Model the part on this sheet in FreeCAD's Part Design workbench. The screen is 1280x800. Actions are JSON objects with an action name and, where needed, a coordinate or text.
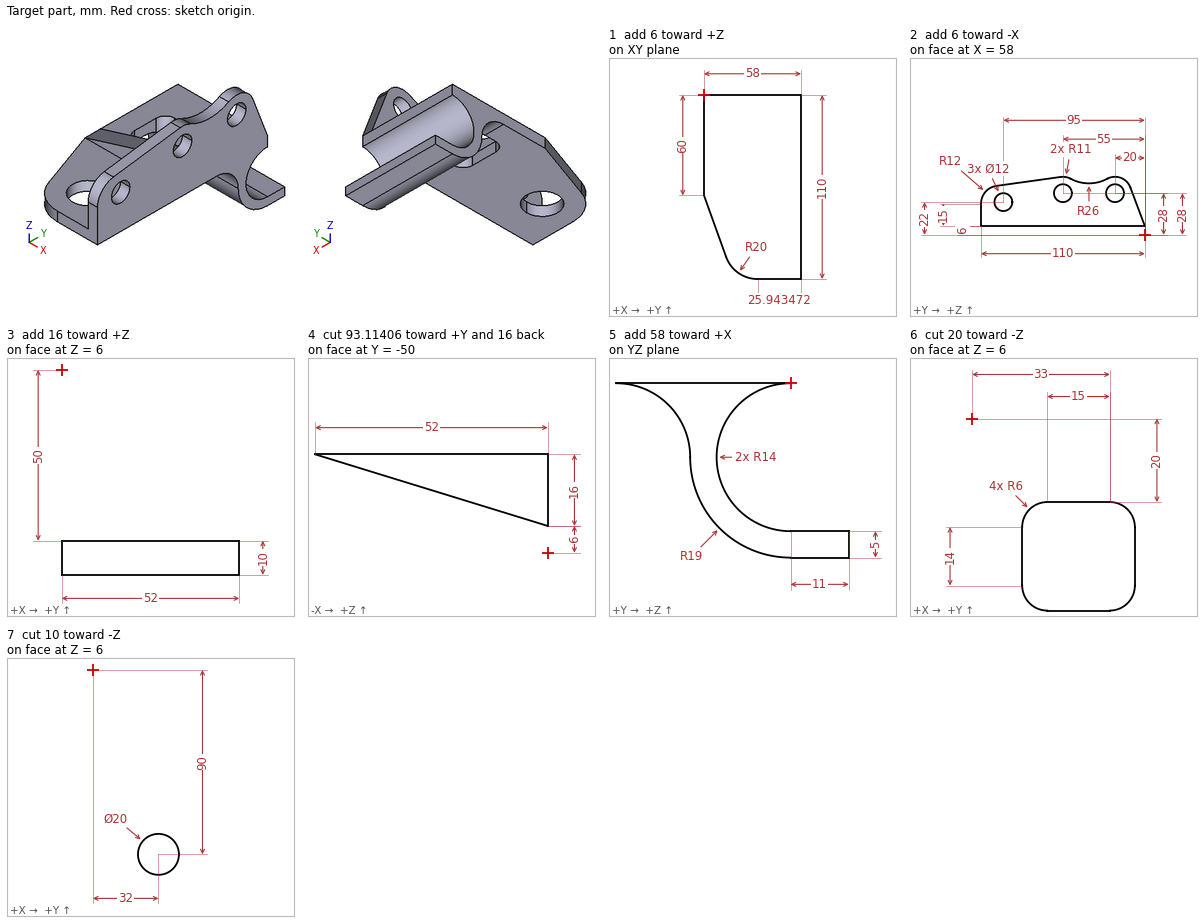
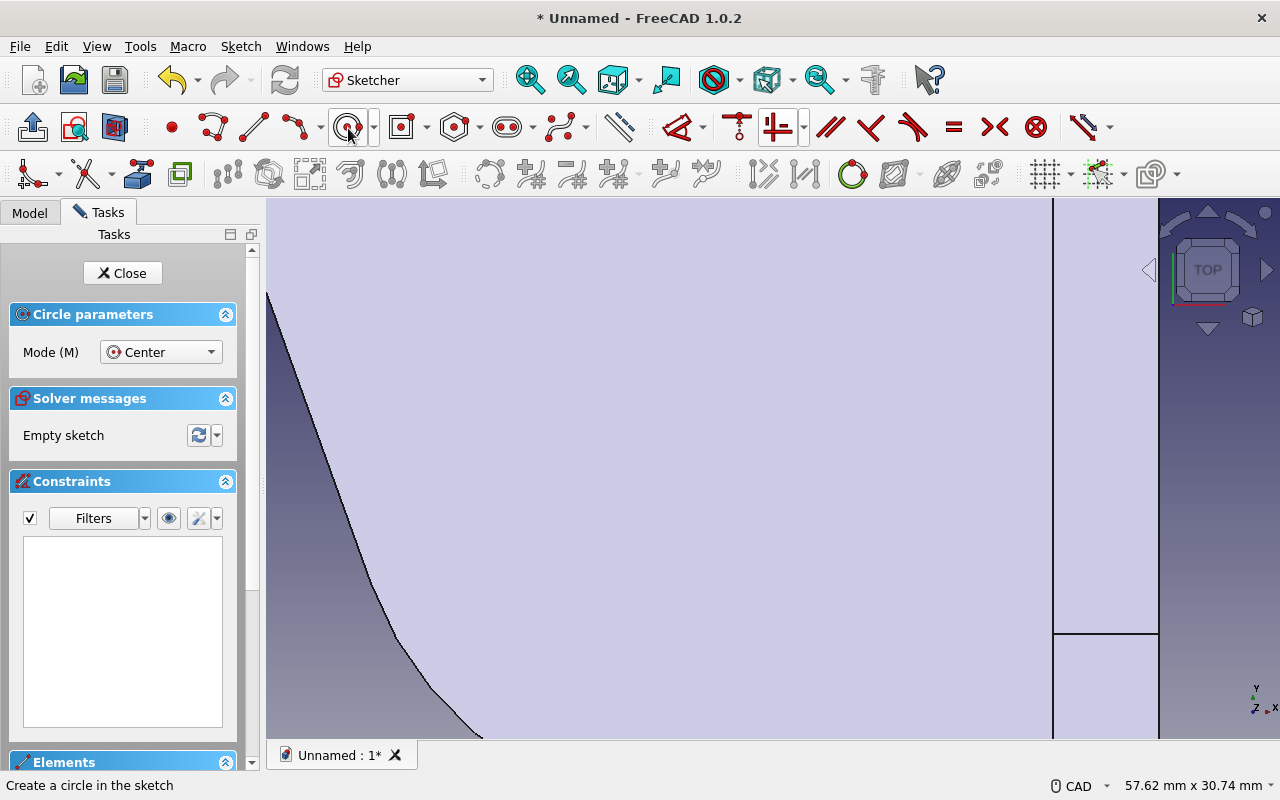
{"action": "left_click", "coordinate": [701, 464]}
{"action": "mouse_move", "coordinate": [826, 340]}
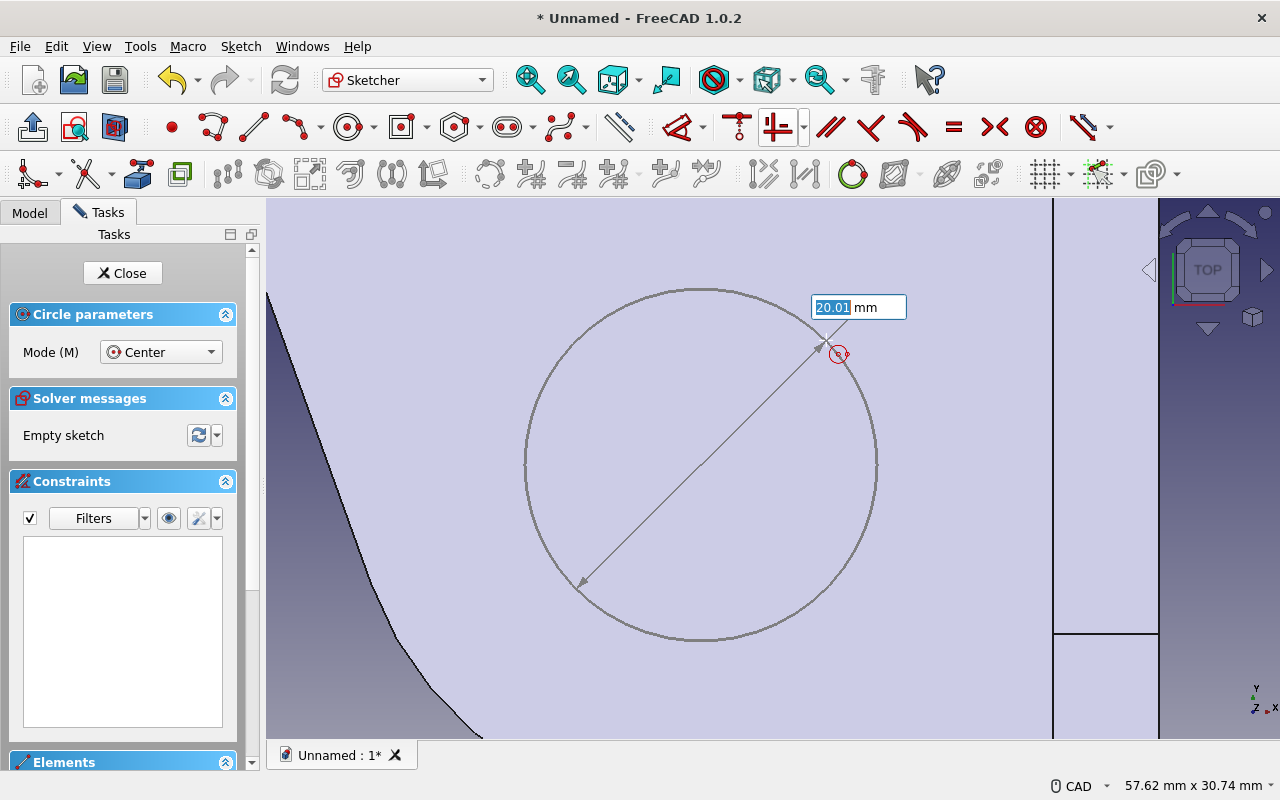
{"action": "type", "text": "20"}
{"action": "key", "text": "Return"}
{"action": "key", "text": "Escape"}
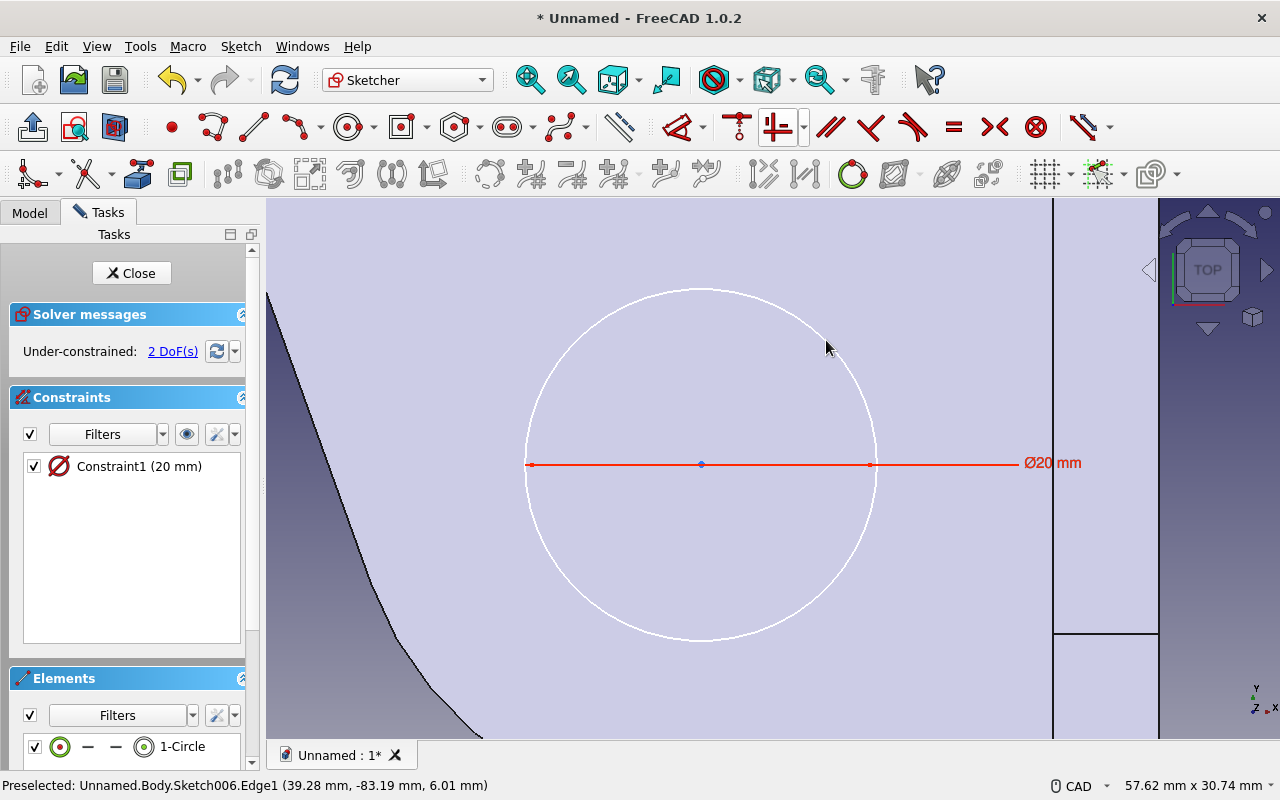
{"action": "key", "text": "d"}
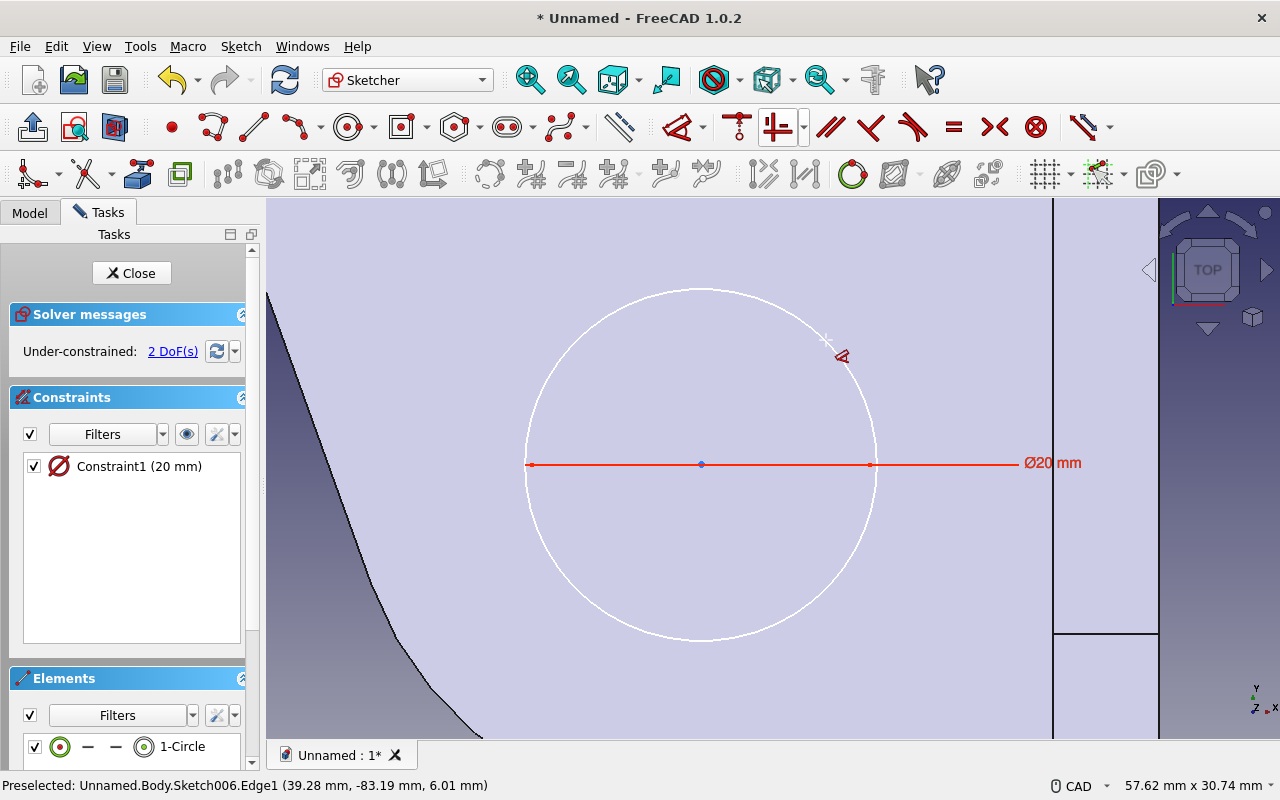
{"action": "left_click", "coordinate": [701, 465]}
{"action": "left_click", "coordinate": [498, 499]}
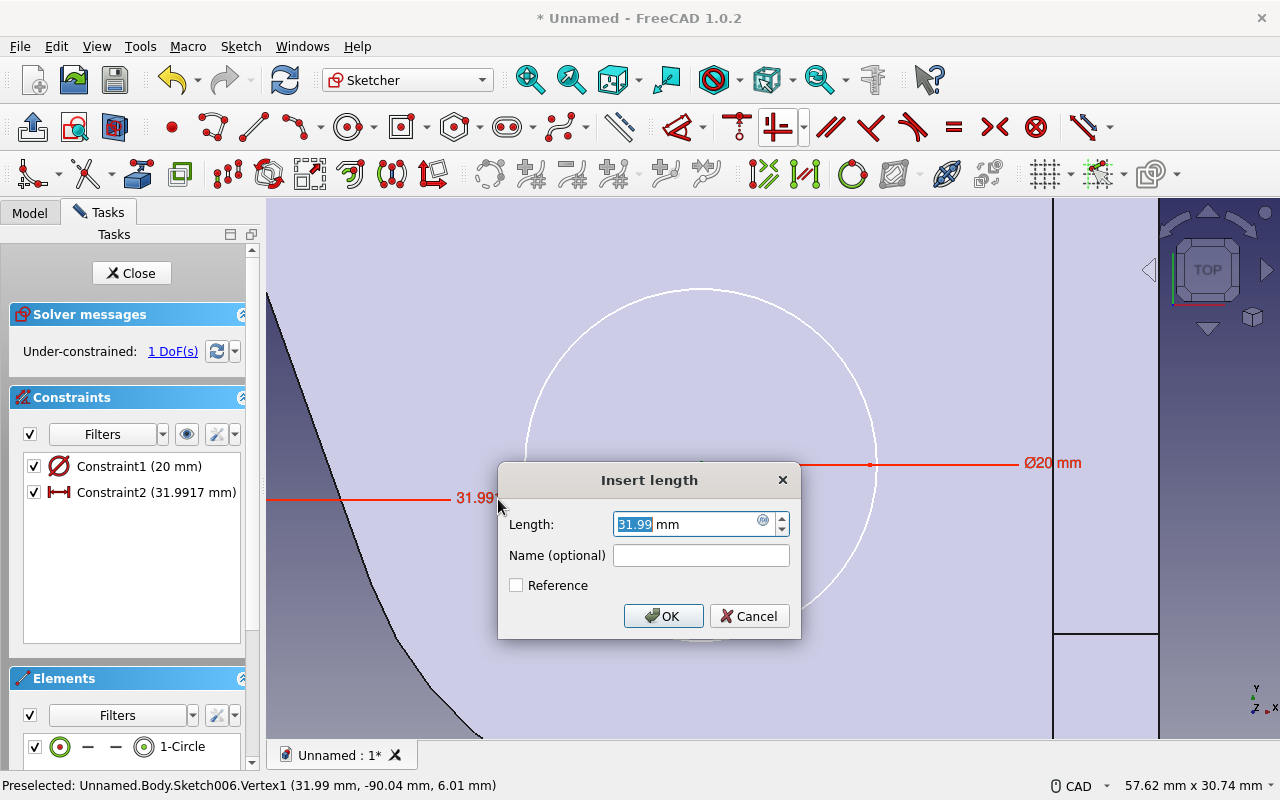
{"action": "type", "text": "32"}
{"action": "key", "text": "Return"}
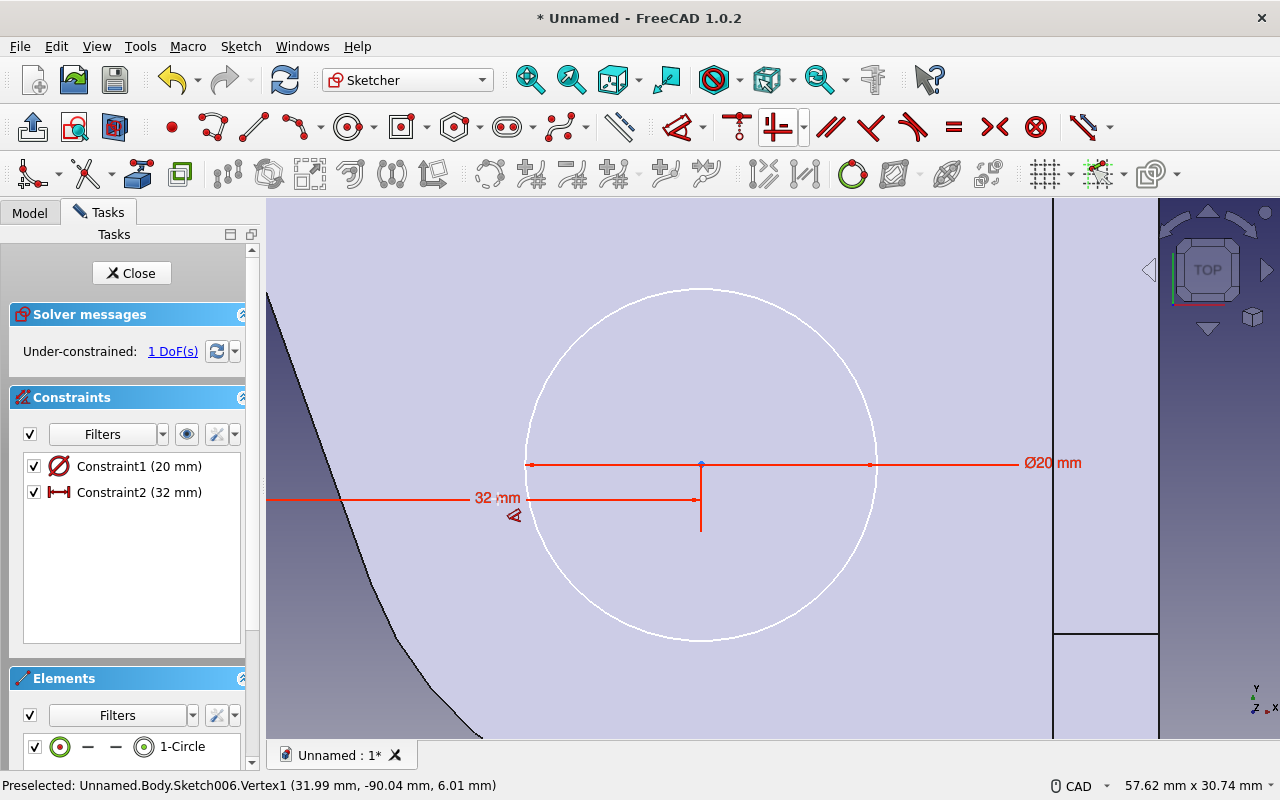
{"action": "left_click", "coordinate": [701, 465]}
{"action": "left_click", "coordinate": [735, 345]}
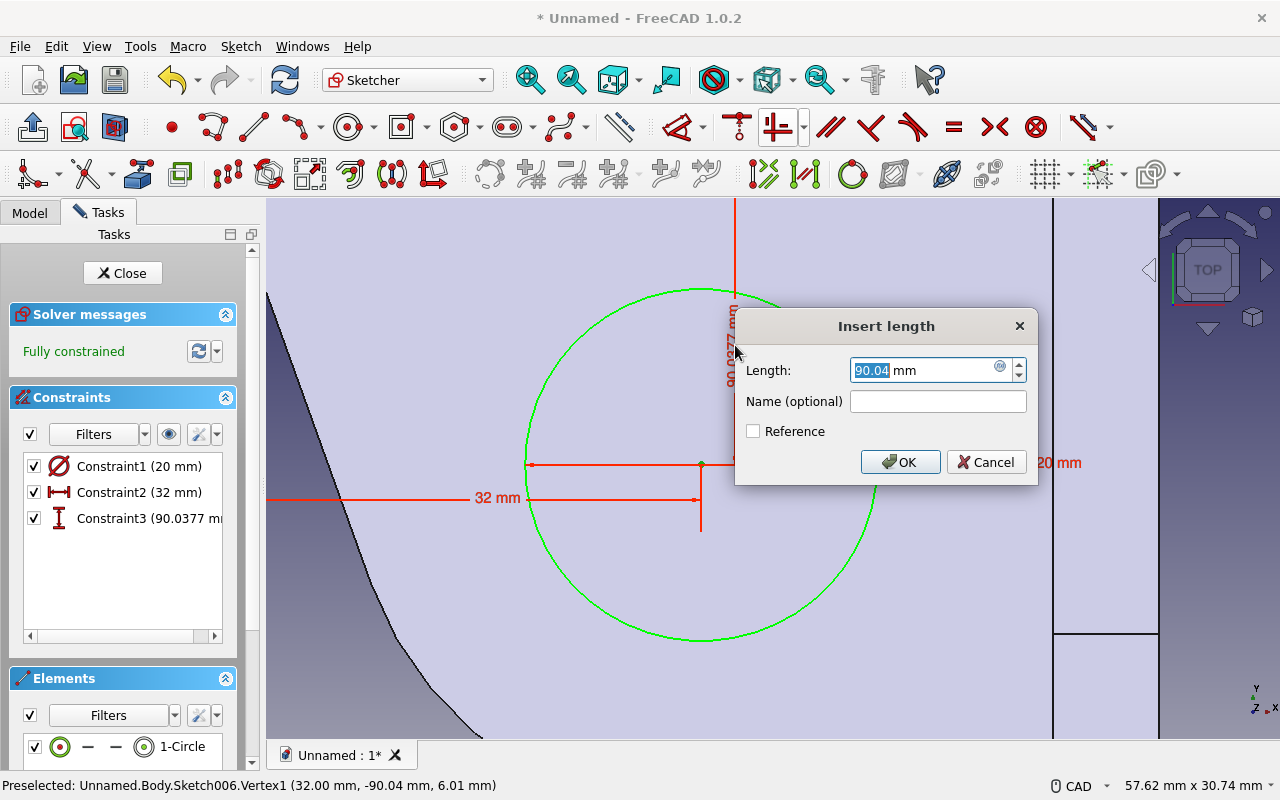
{"action": "type", "text": "90"}
{"action": "key", "text": "Return"}
{"action": "key", "text": "Escape"}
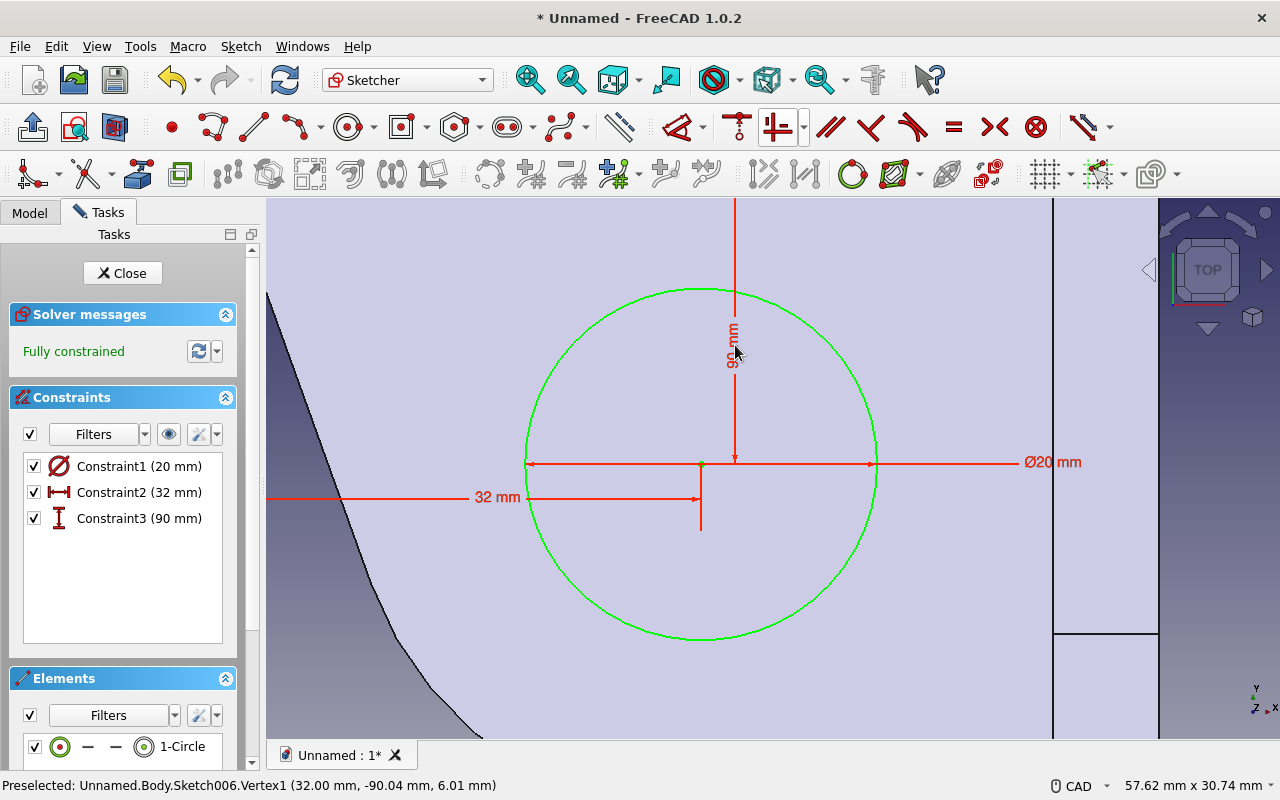
{"action": "left_click", "coordinate": [123, 273]}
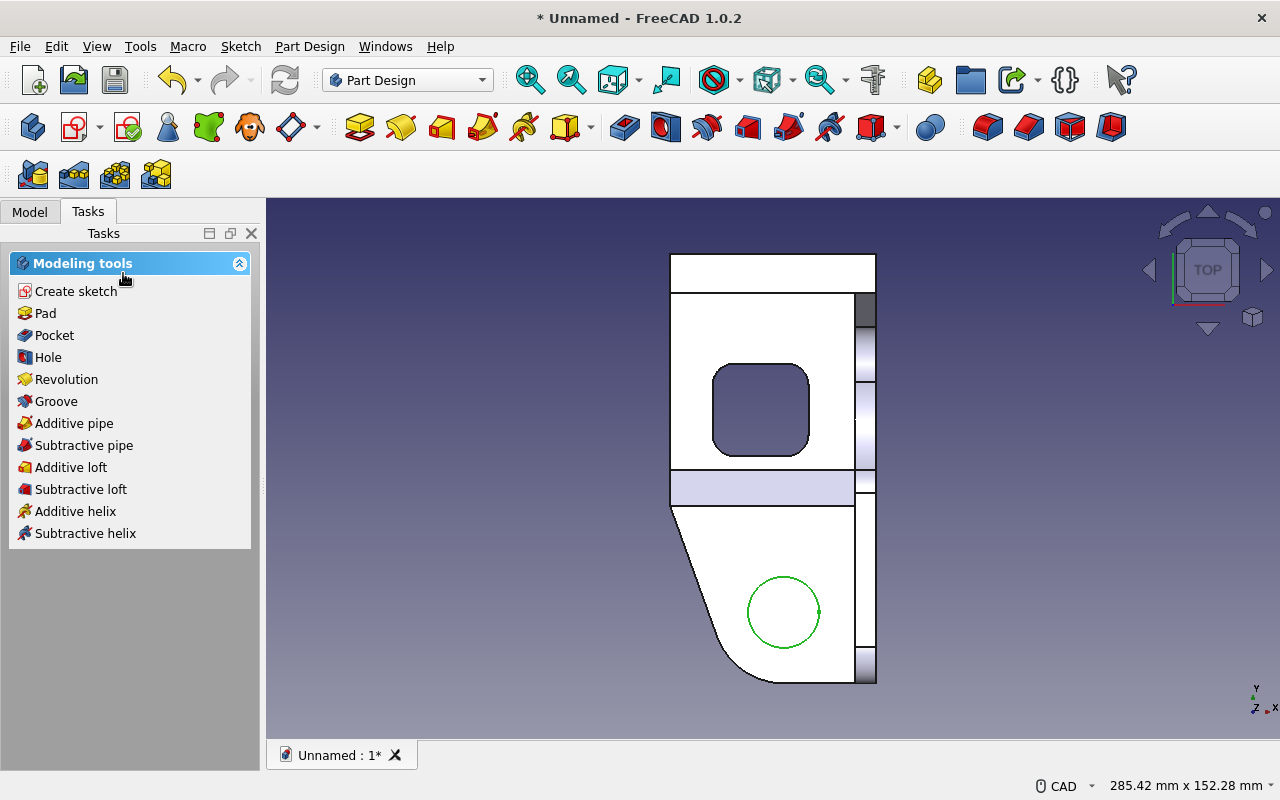
{"action": "left_click", "coordinate": [625, 128]}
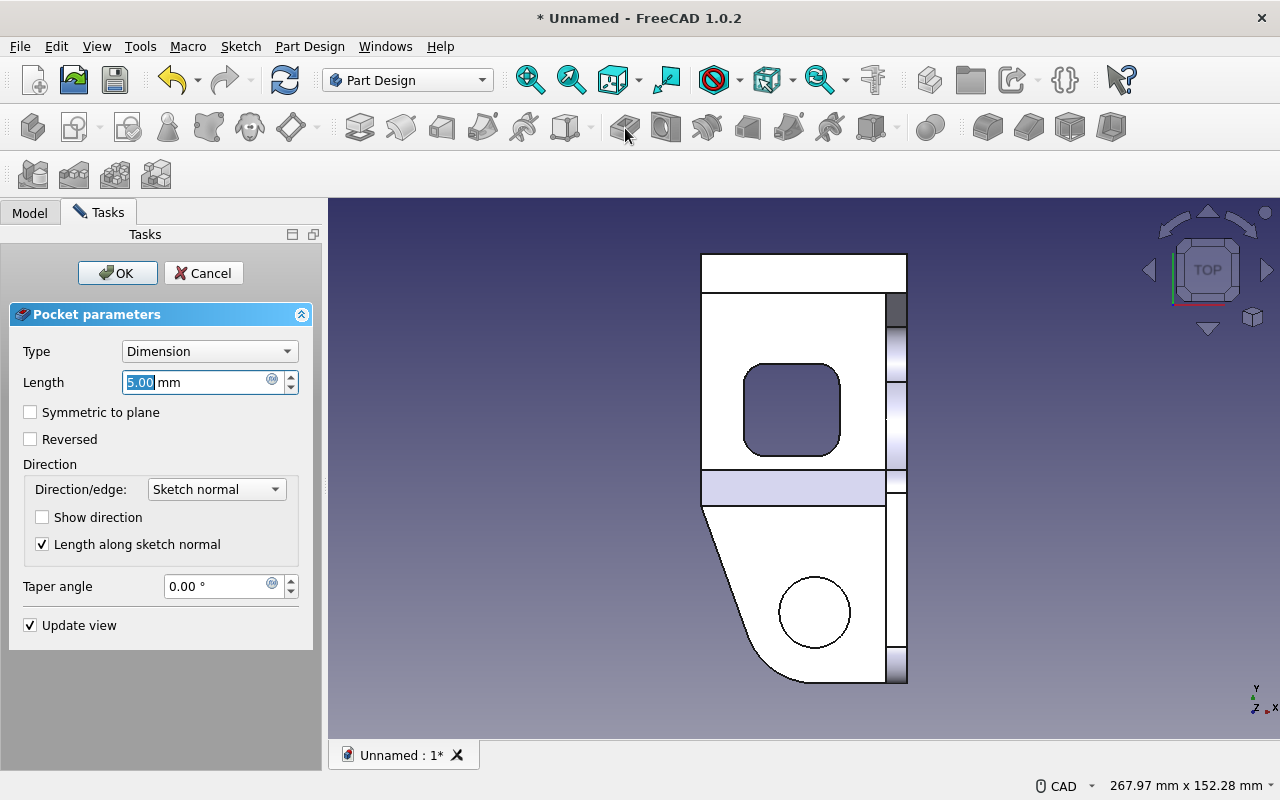
{"action": "type", "text": "10"}
{"action": "key", "text": "Tab"}